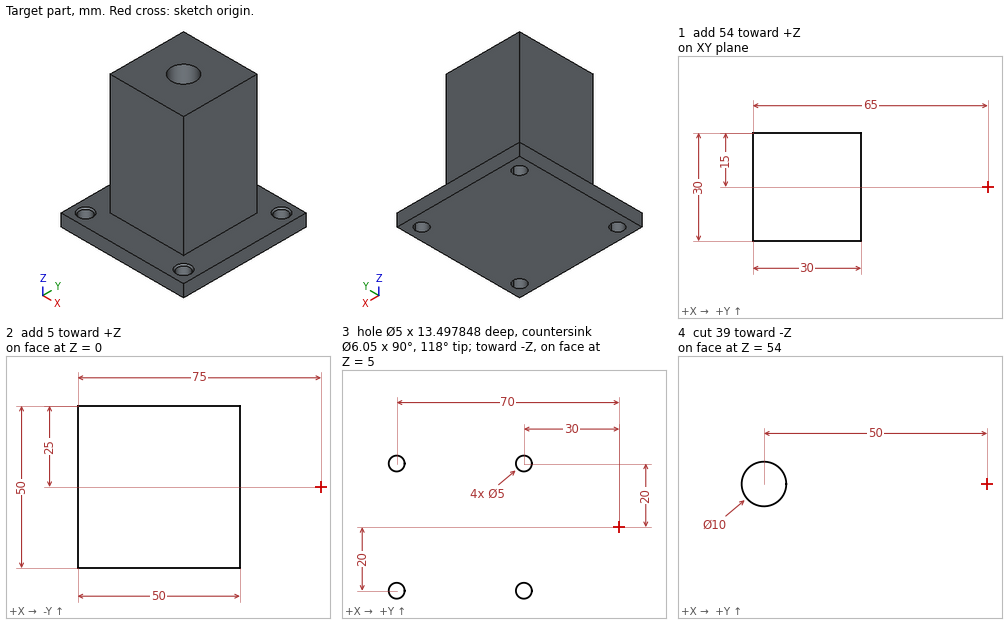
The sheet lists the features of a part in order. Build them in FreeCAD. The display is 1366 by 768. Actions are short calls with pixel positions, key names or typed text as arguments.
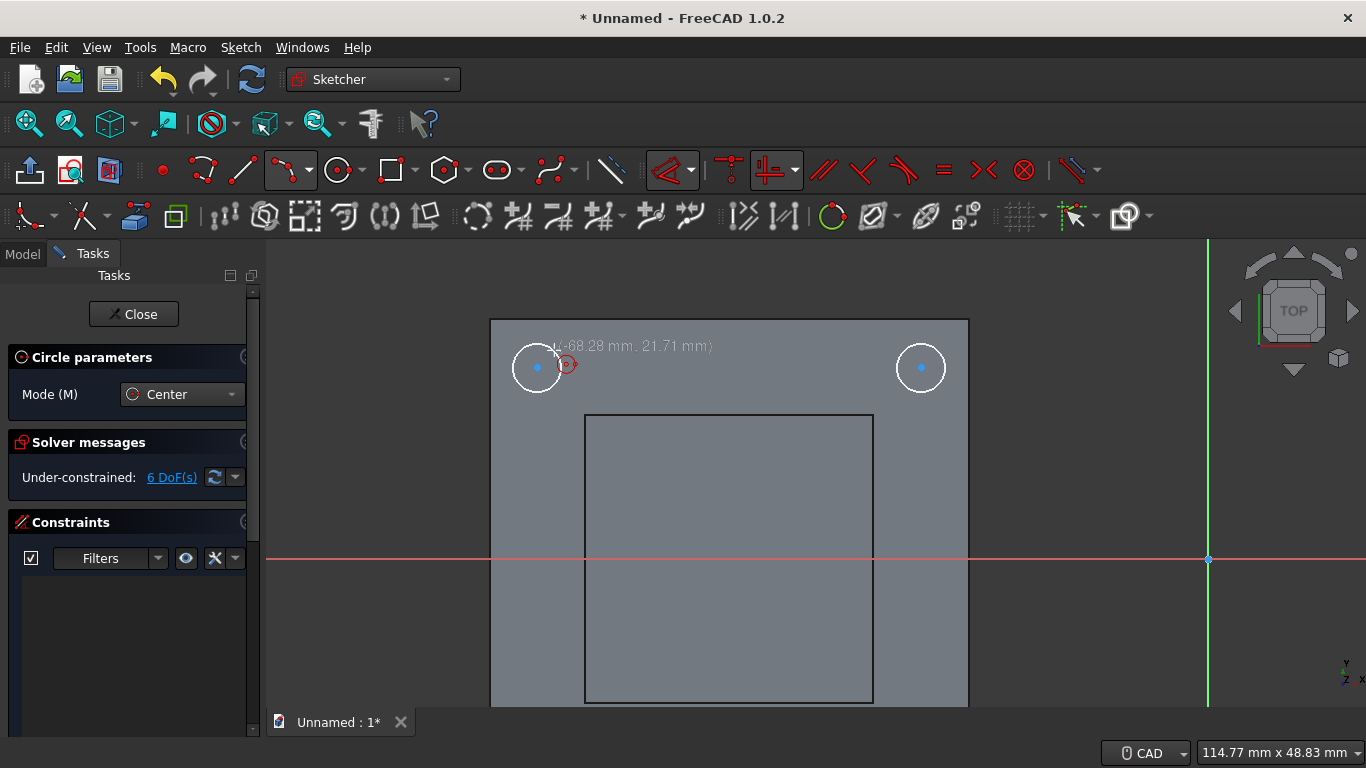
scroll(517, 298, down, 2)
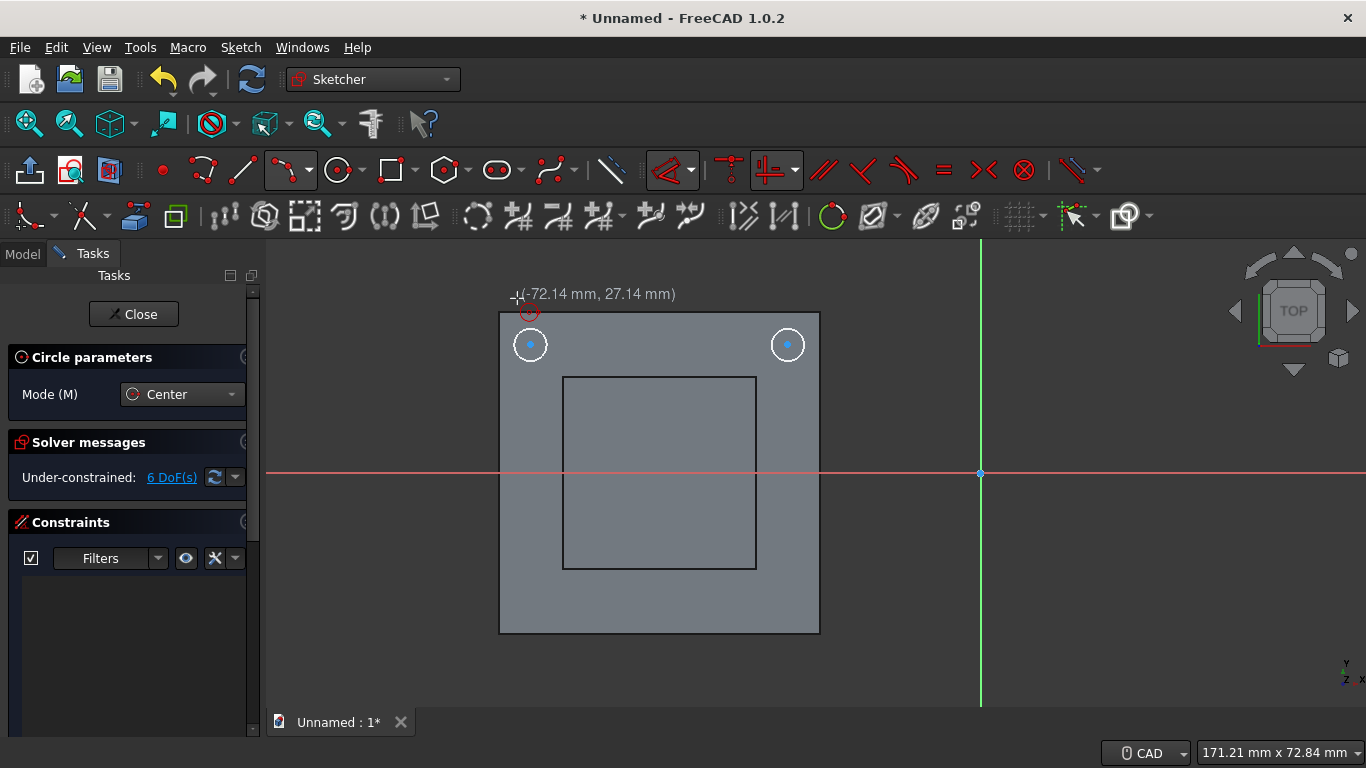
scroll(531, 602, up, 2)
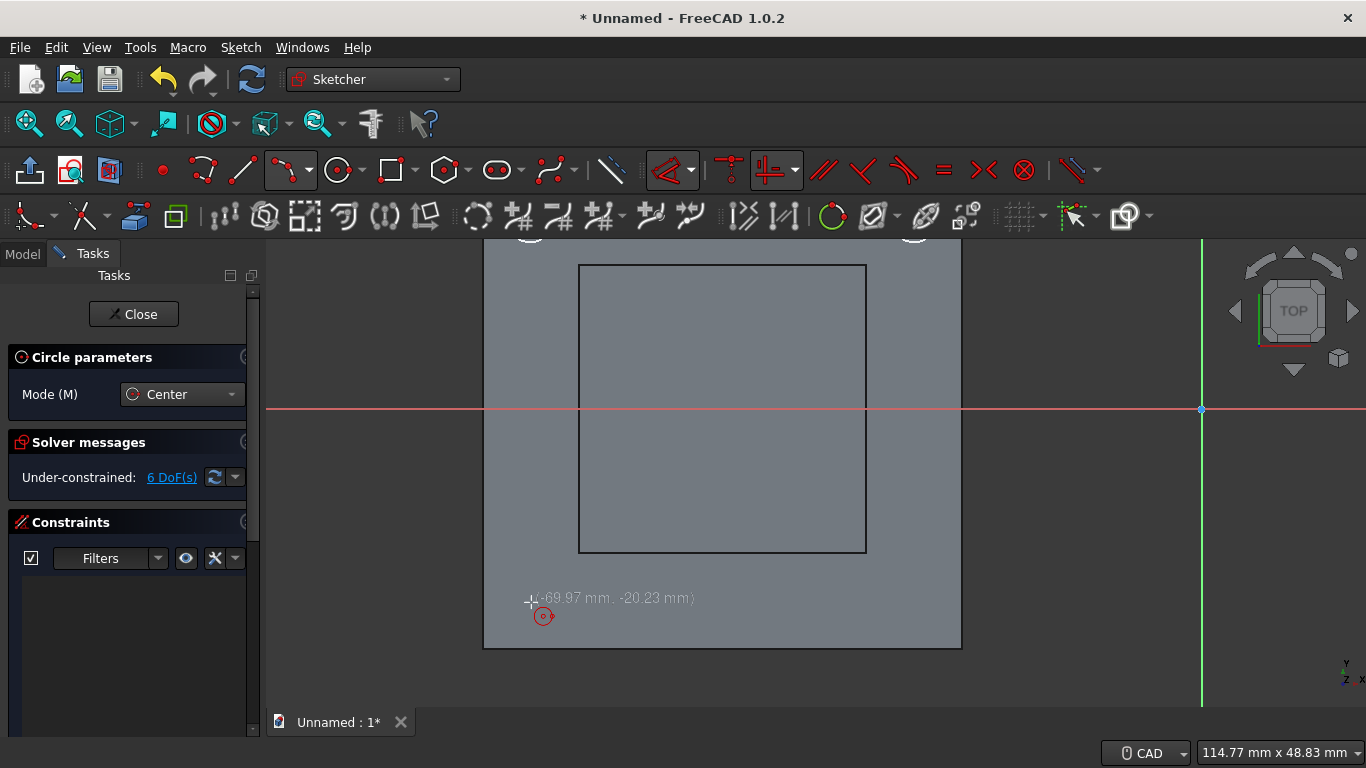
click(531, 601)
click(548, 584)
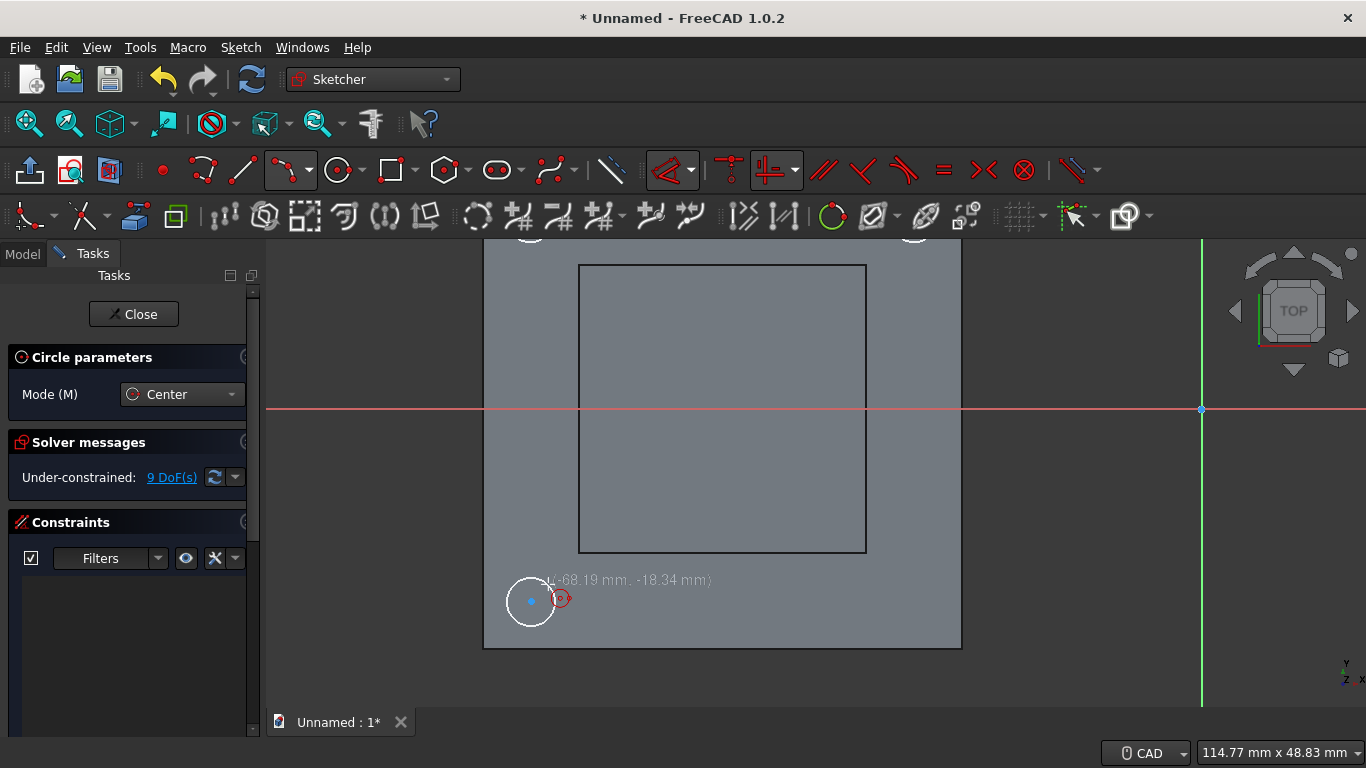
click(914, 601)
click(931, 584)
key(Escape)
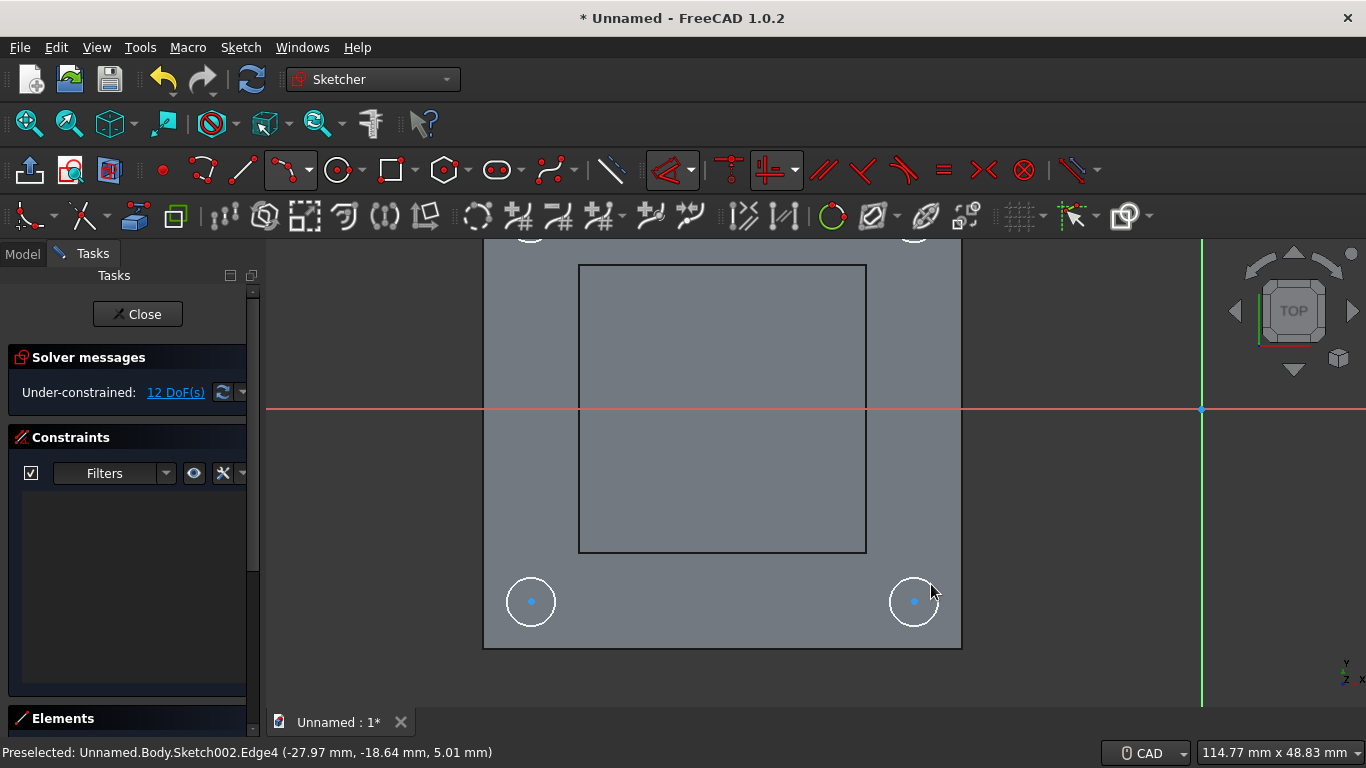
scroll(531, 603, down, 2)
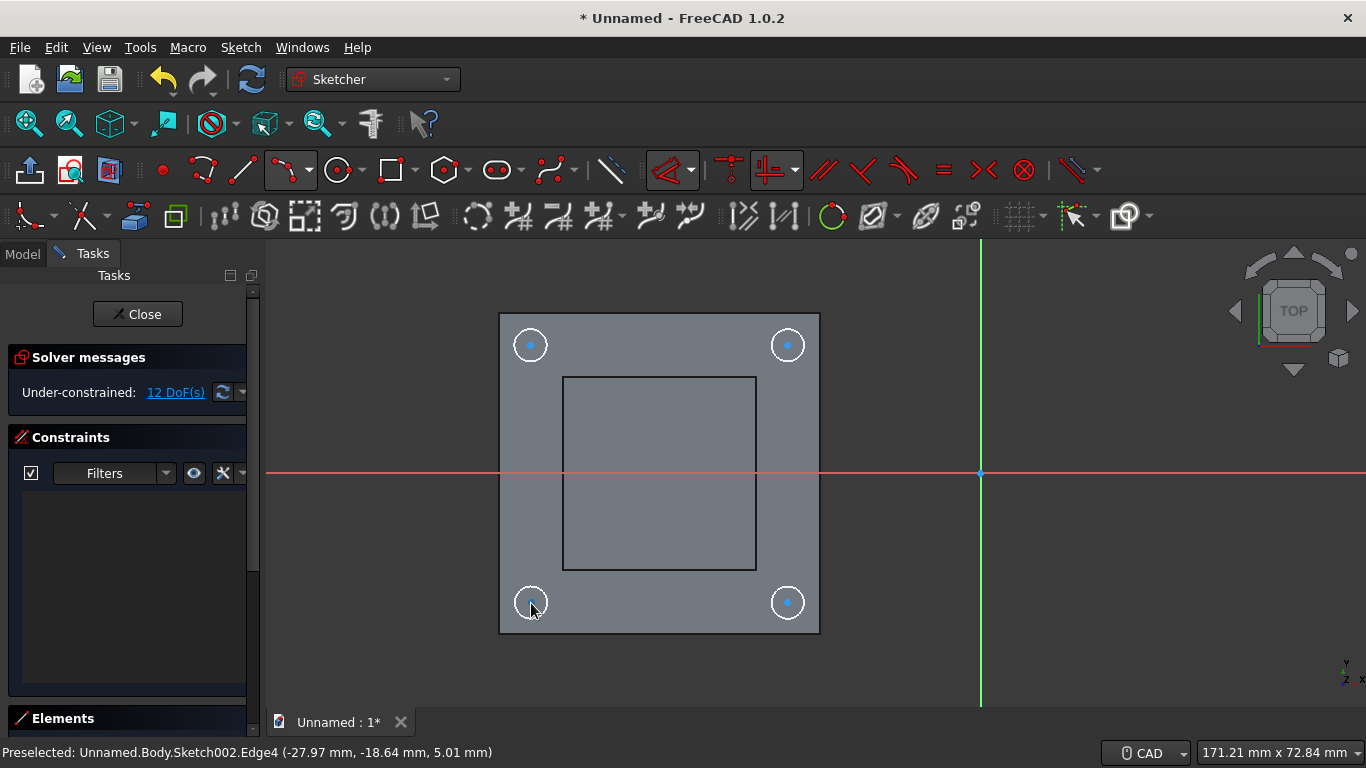
click(799, 334)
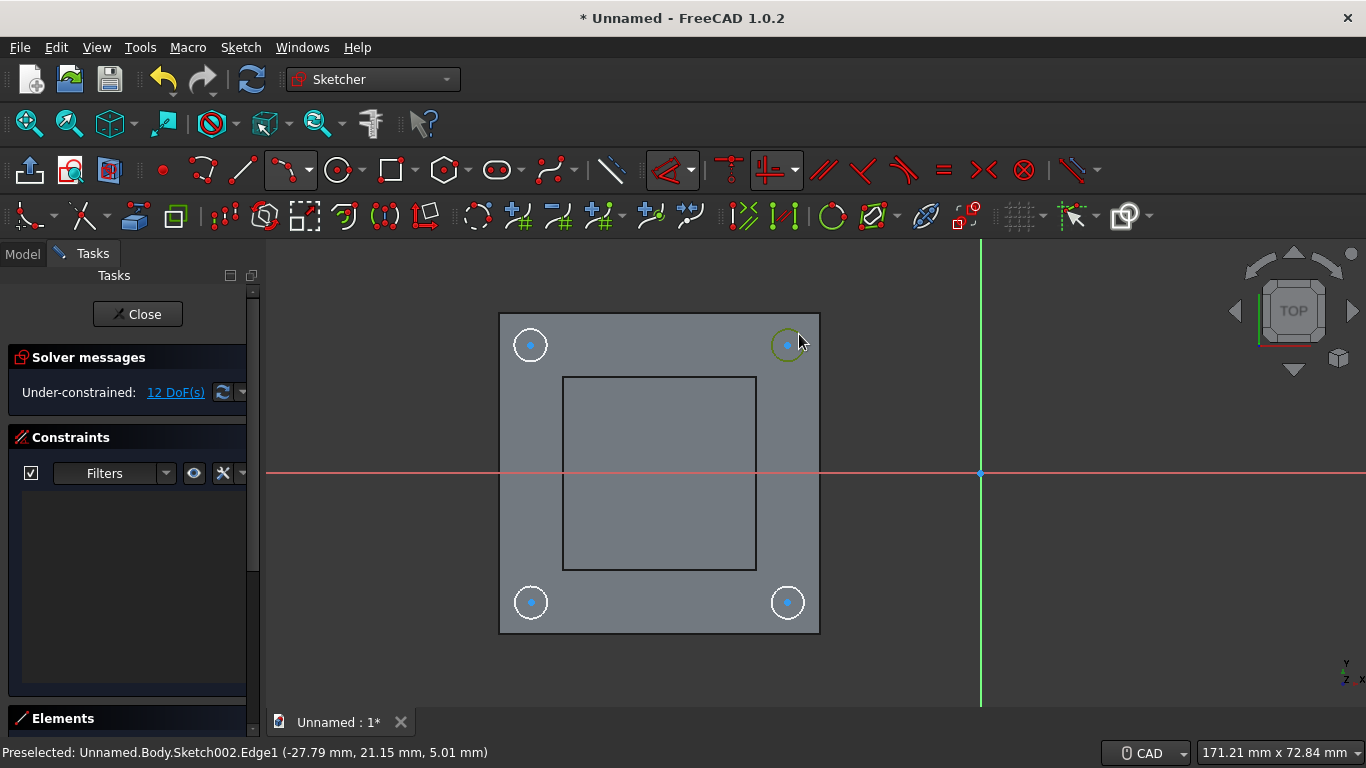
click(542, 334)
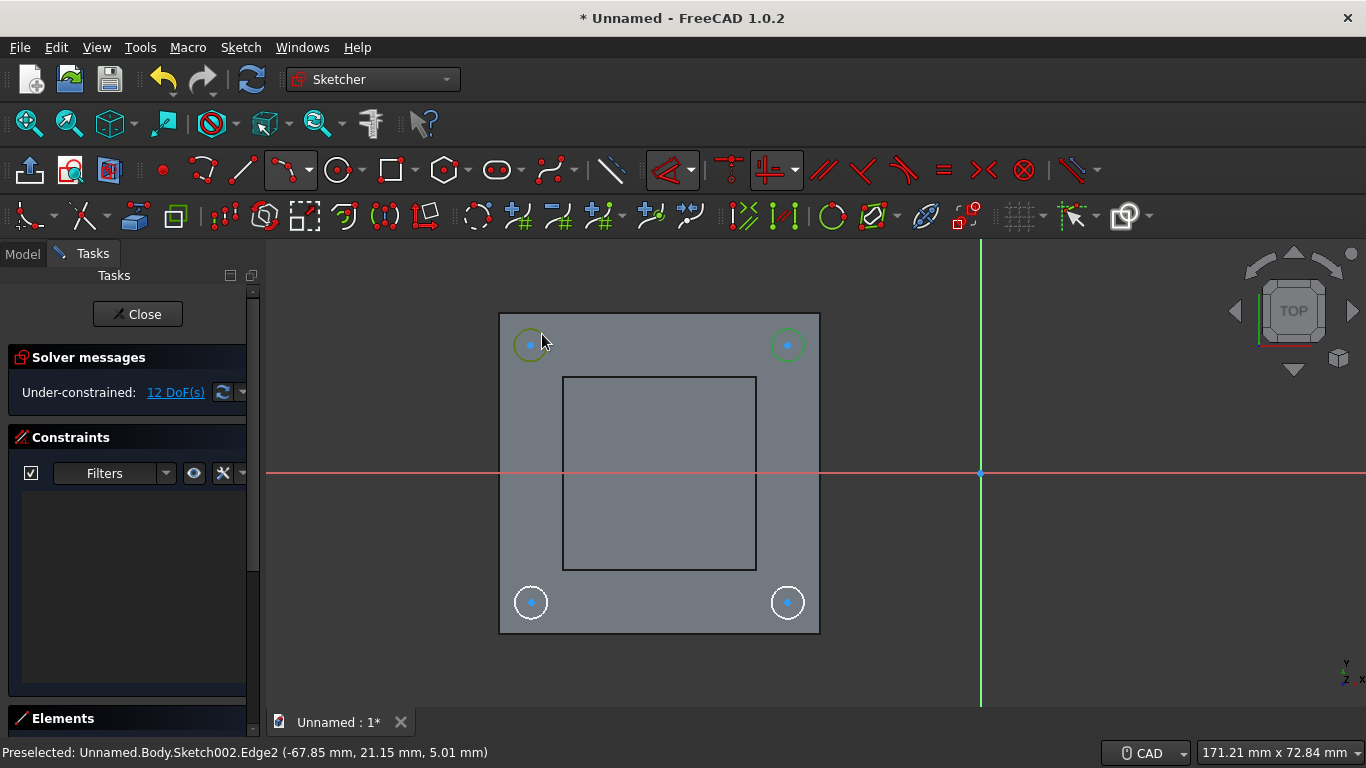
click(542, 591)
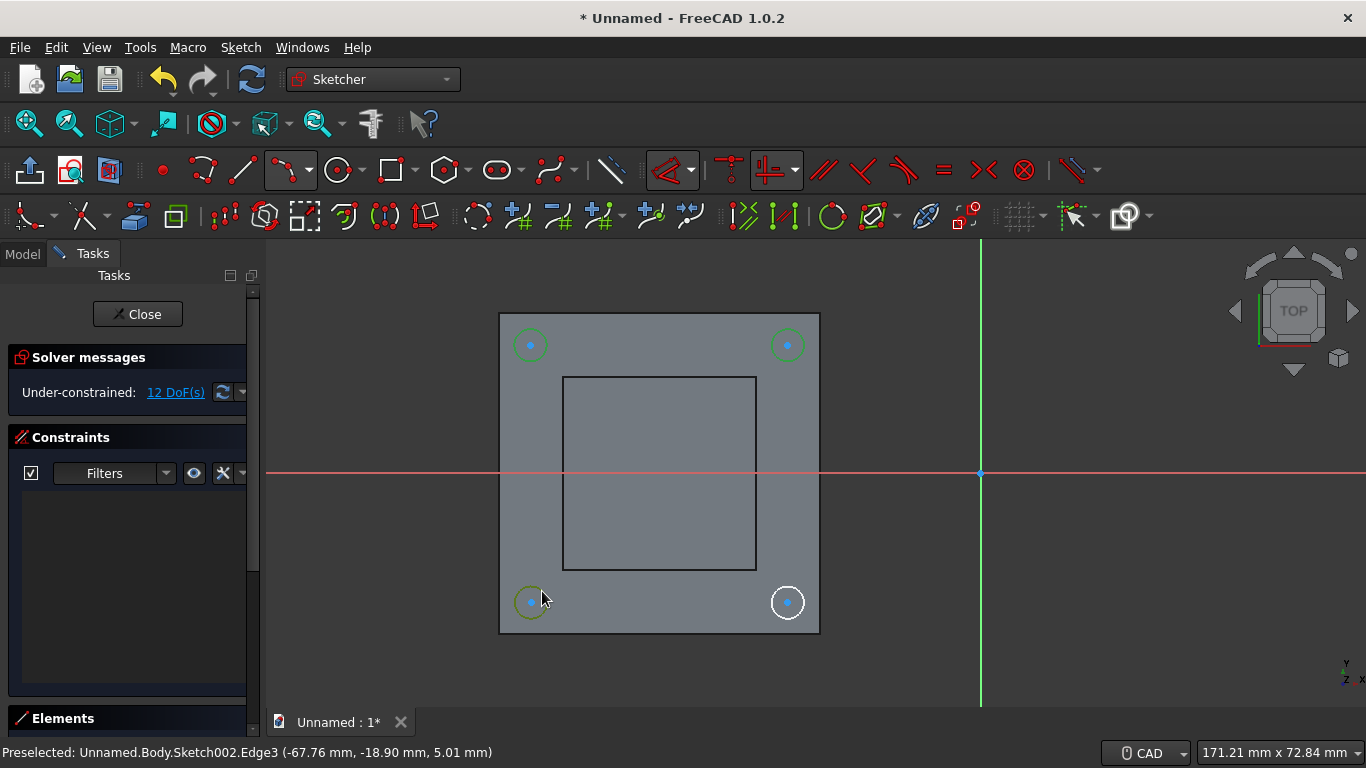
click(799, 591)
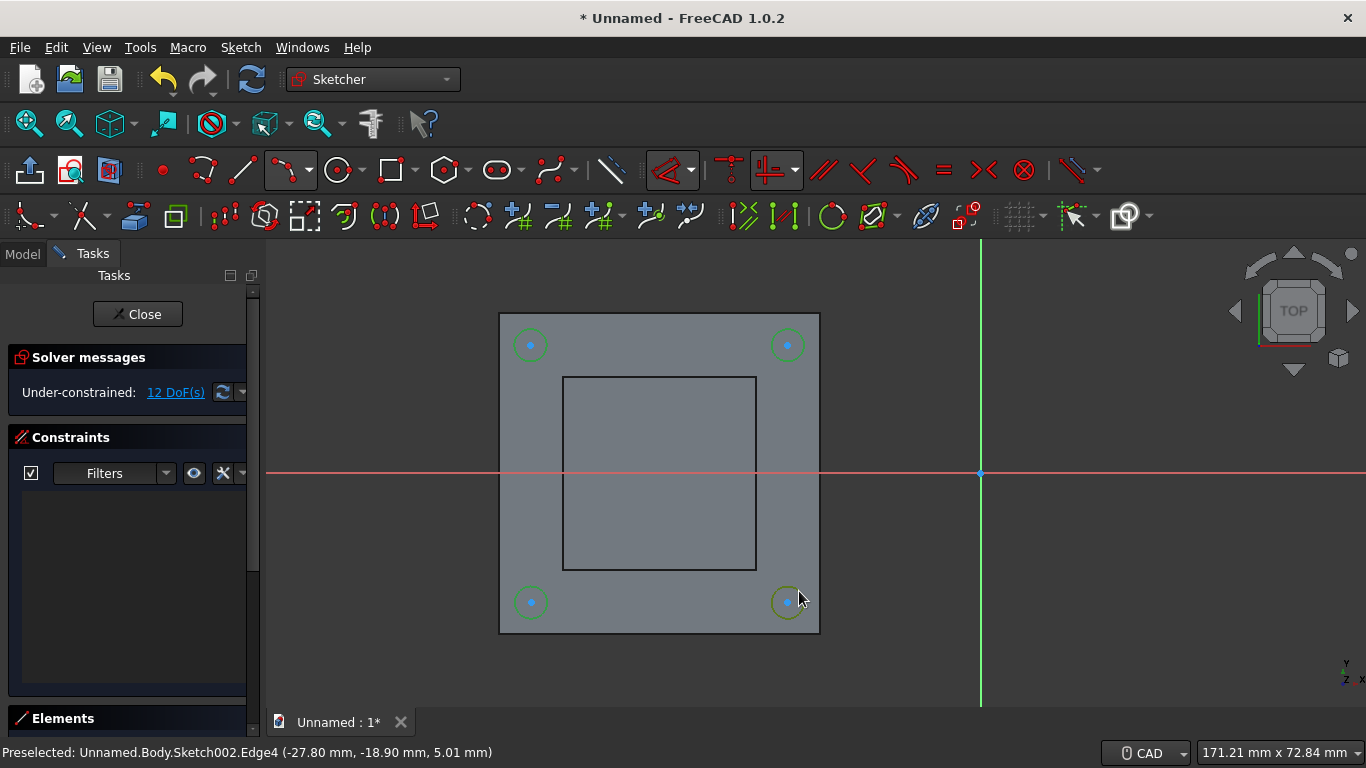
key(e)